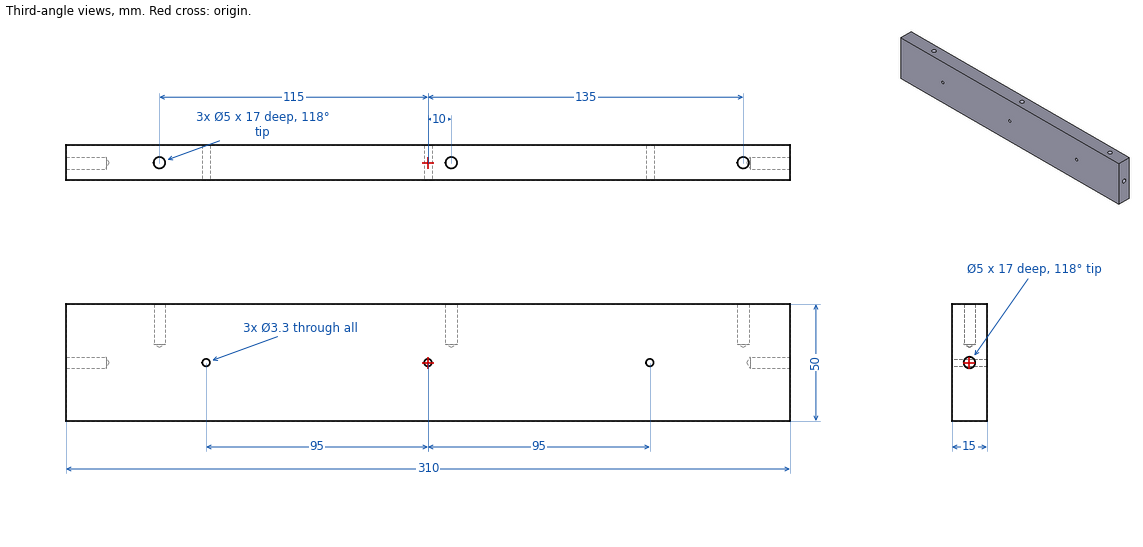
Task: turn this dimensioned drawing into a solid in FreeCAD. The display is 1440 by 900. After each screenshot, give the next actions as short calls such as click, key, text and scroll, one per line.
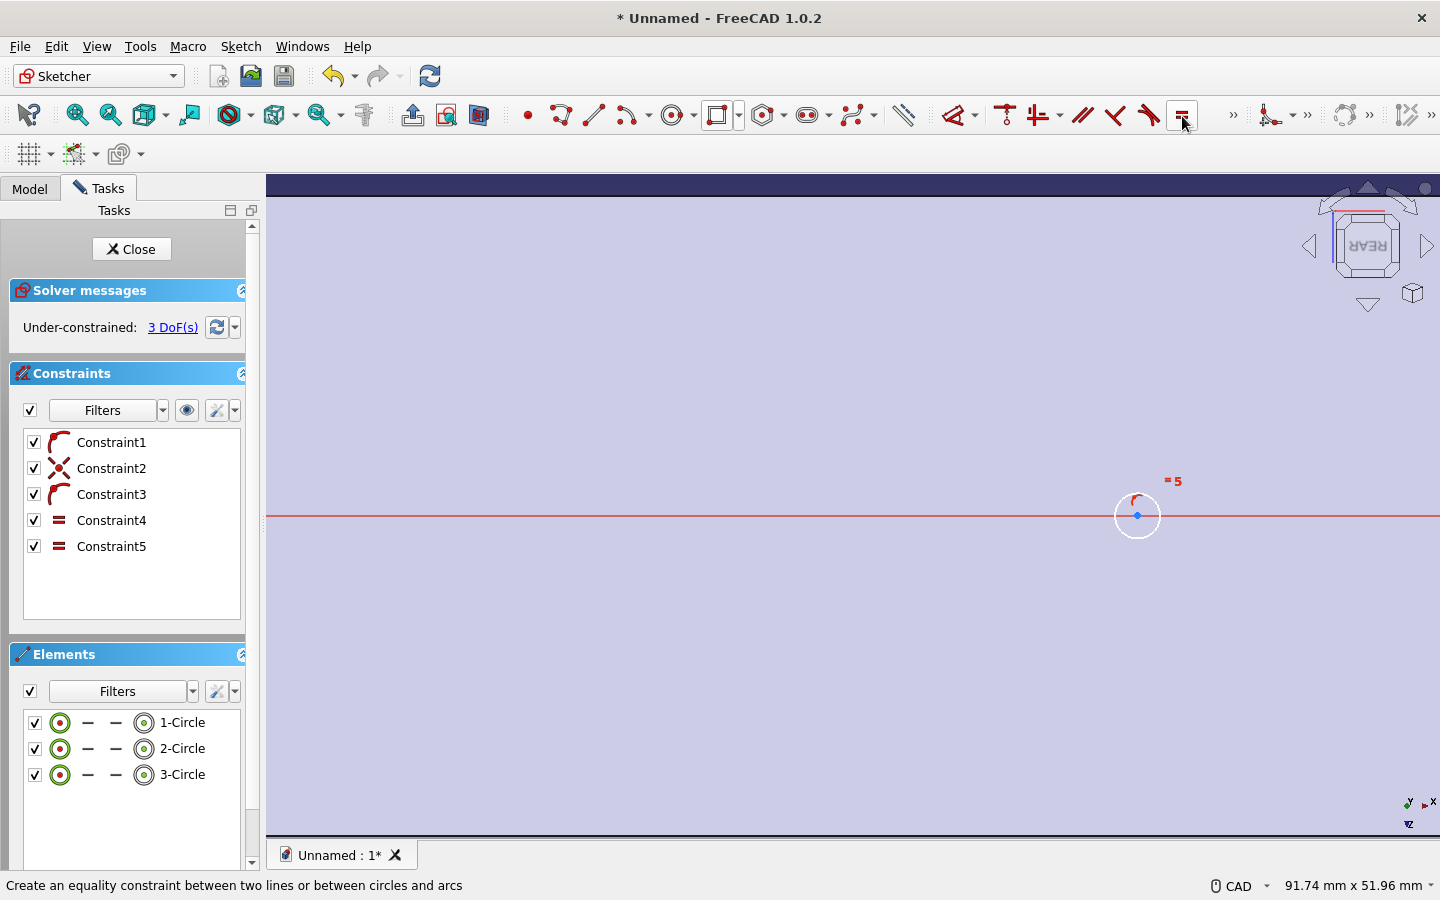
click(952, 116)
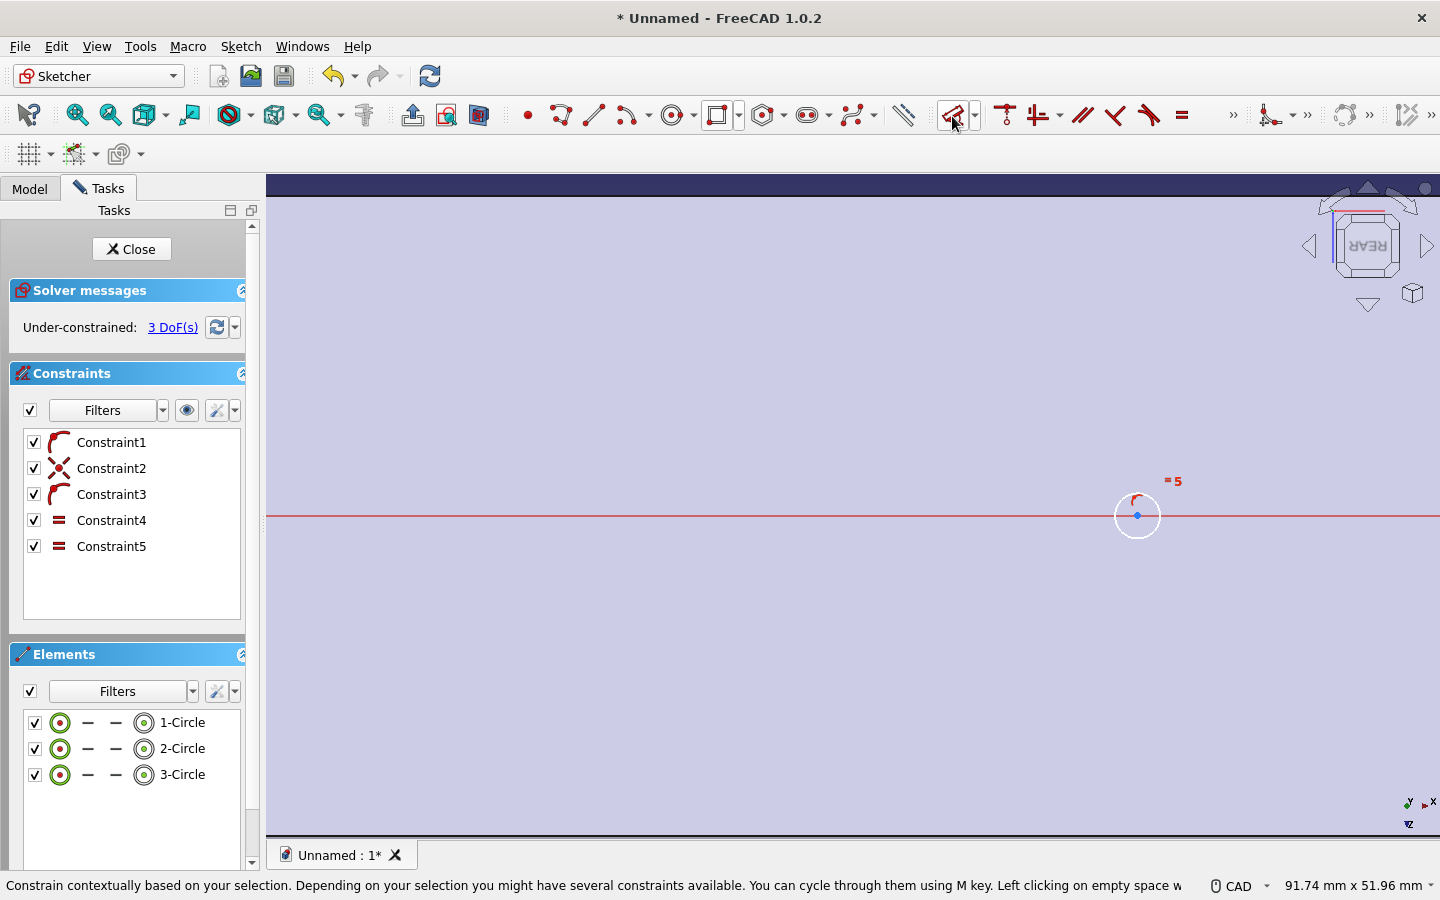
scroll(1156, 502, down, 6)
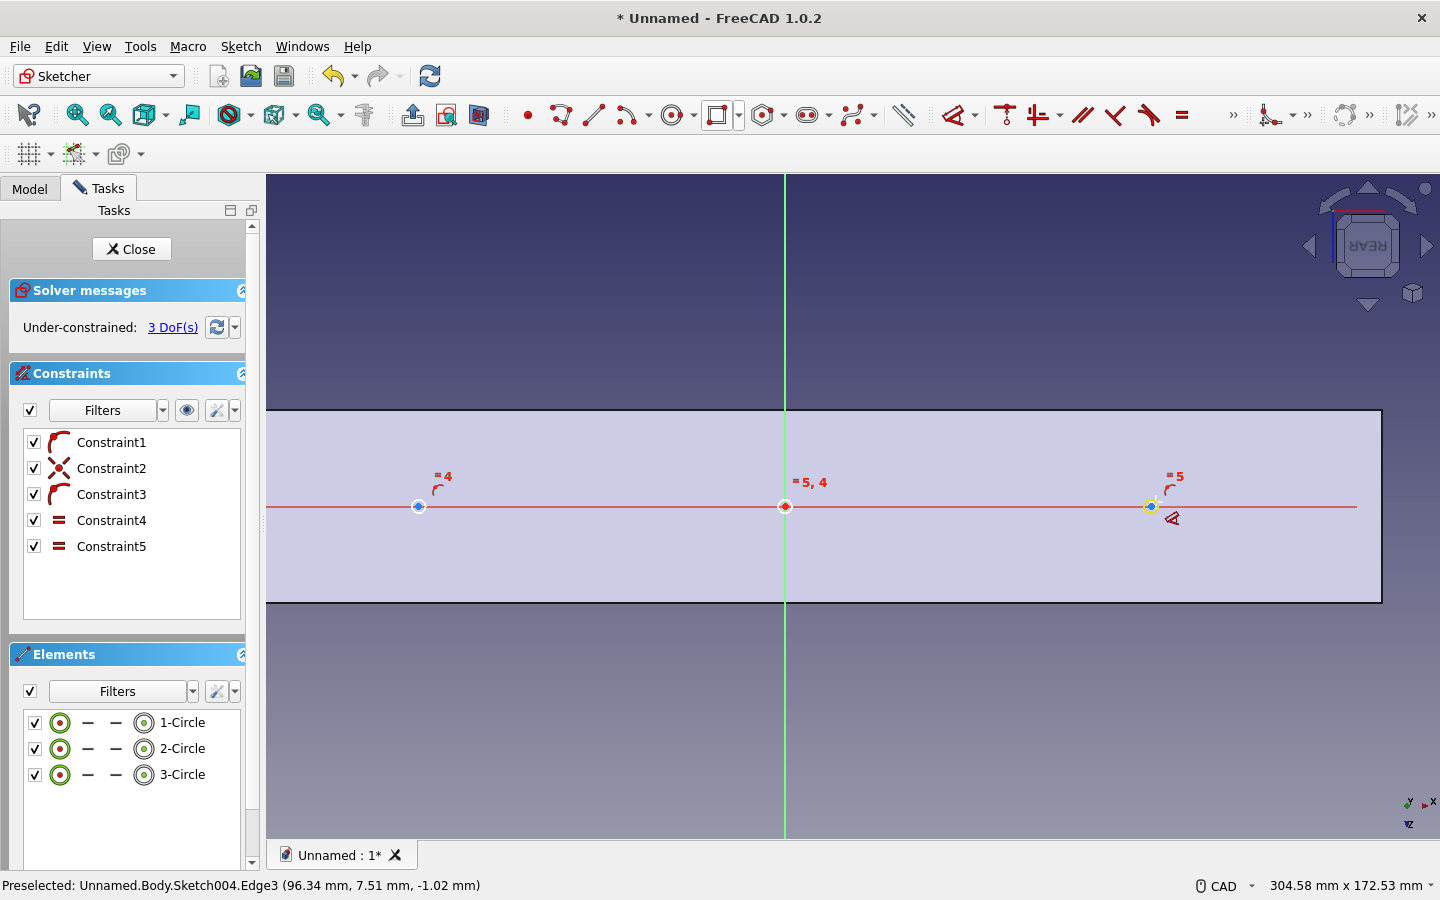
scroll(424, 502, up, 6)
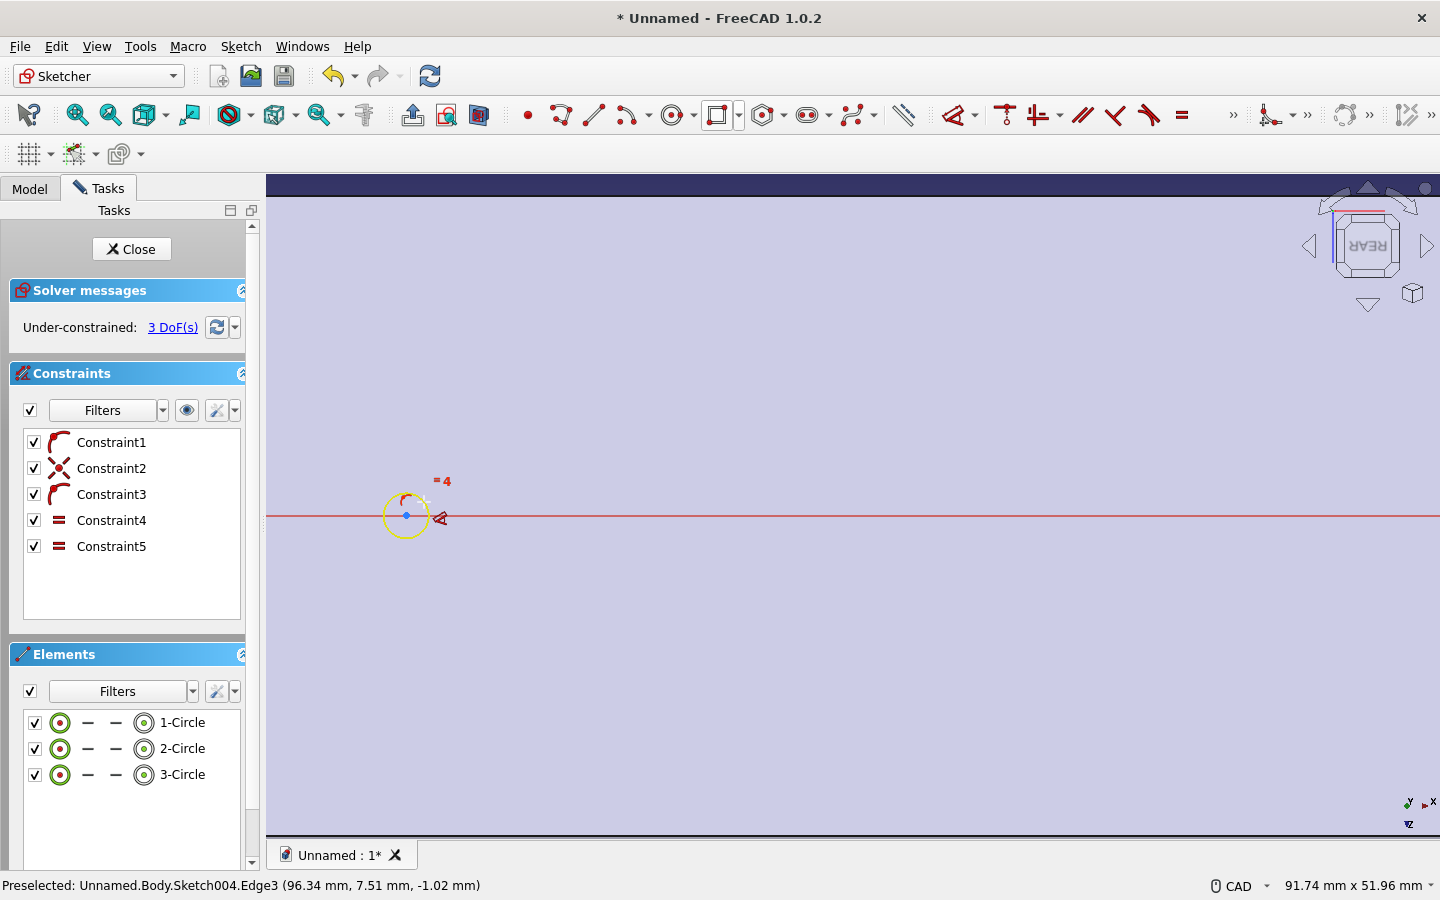
click(422, 500)
click(444, 477)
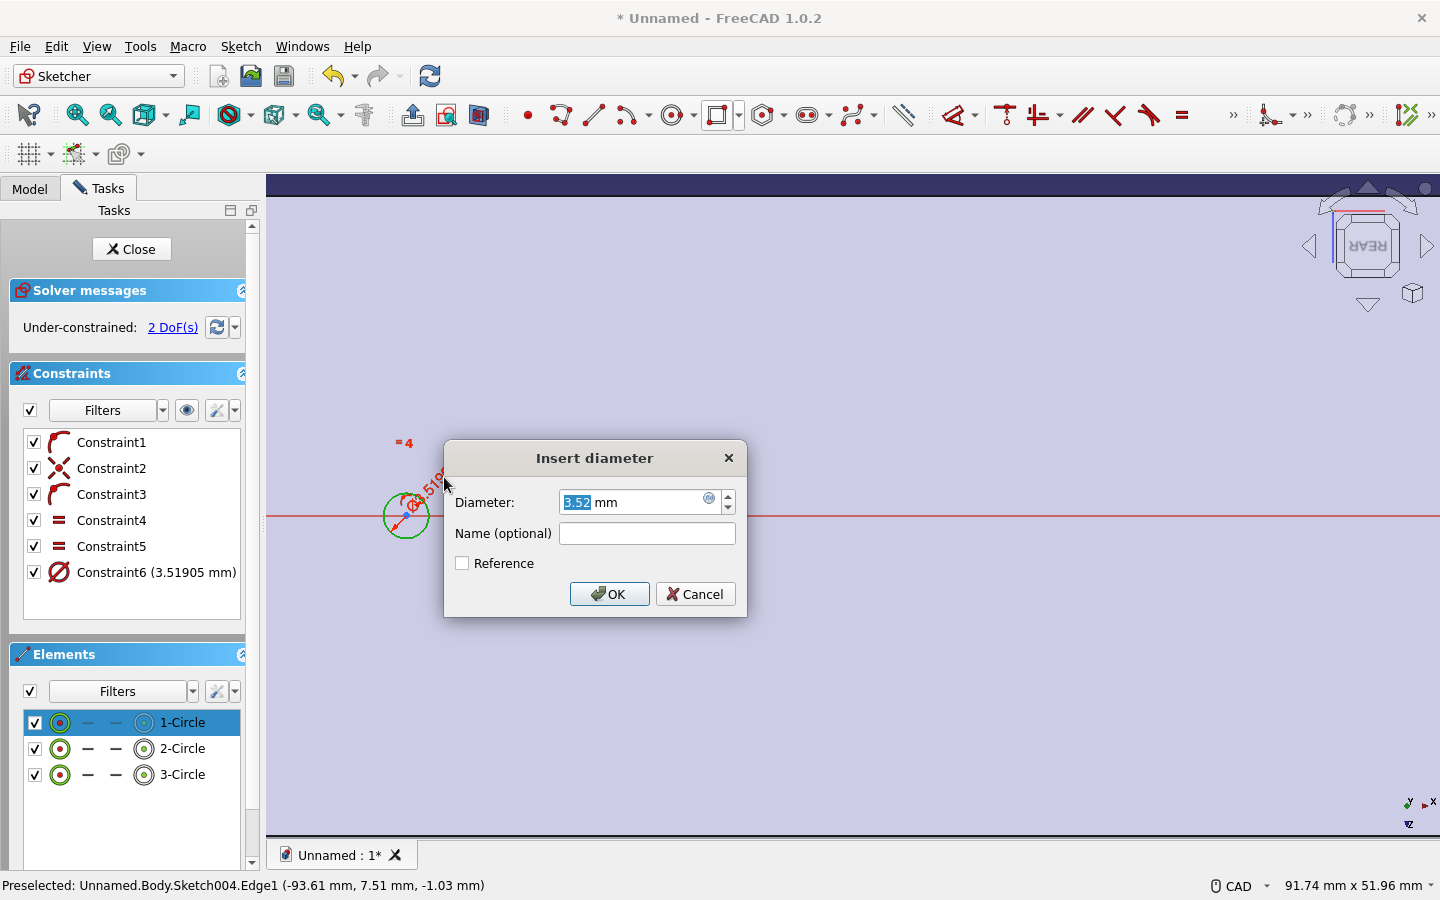
text(3.3)
key(Return)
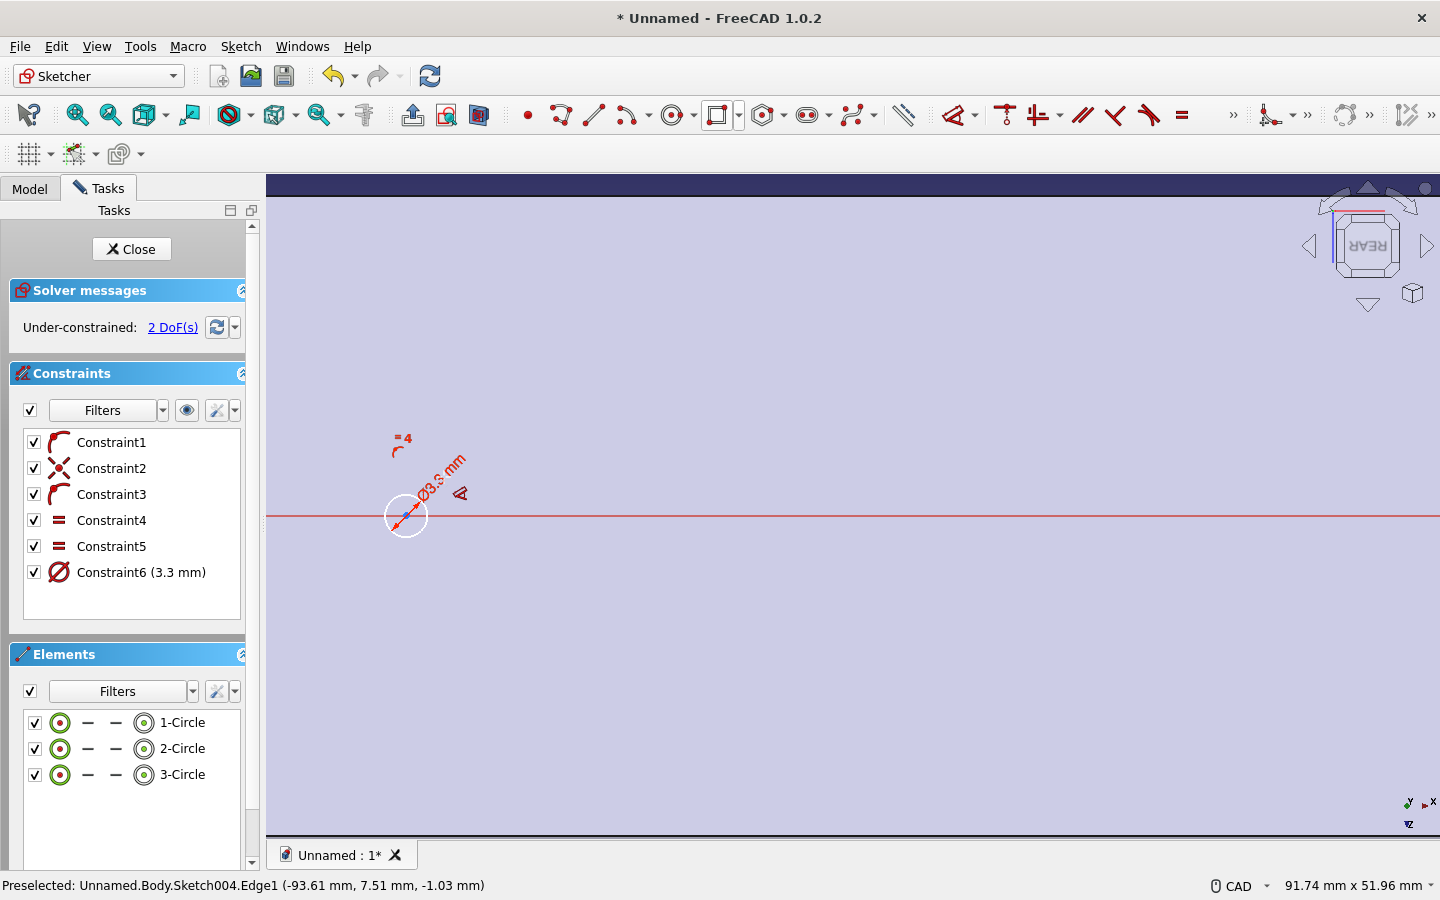
click(406, 516)
click(841, 550)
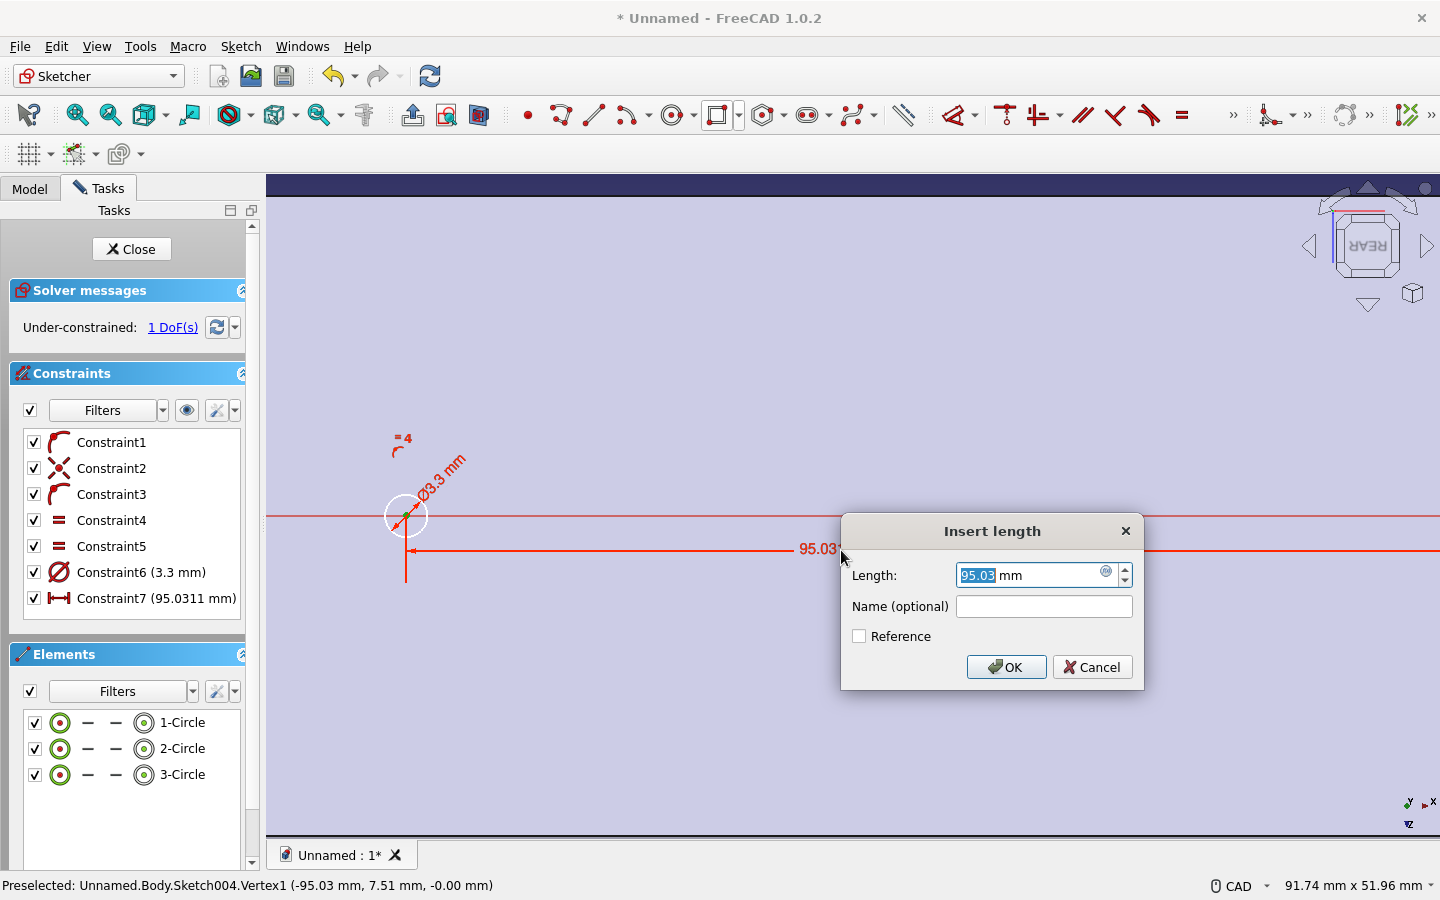
text(95)
key(Return)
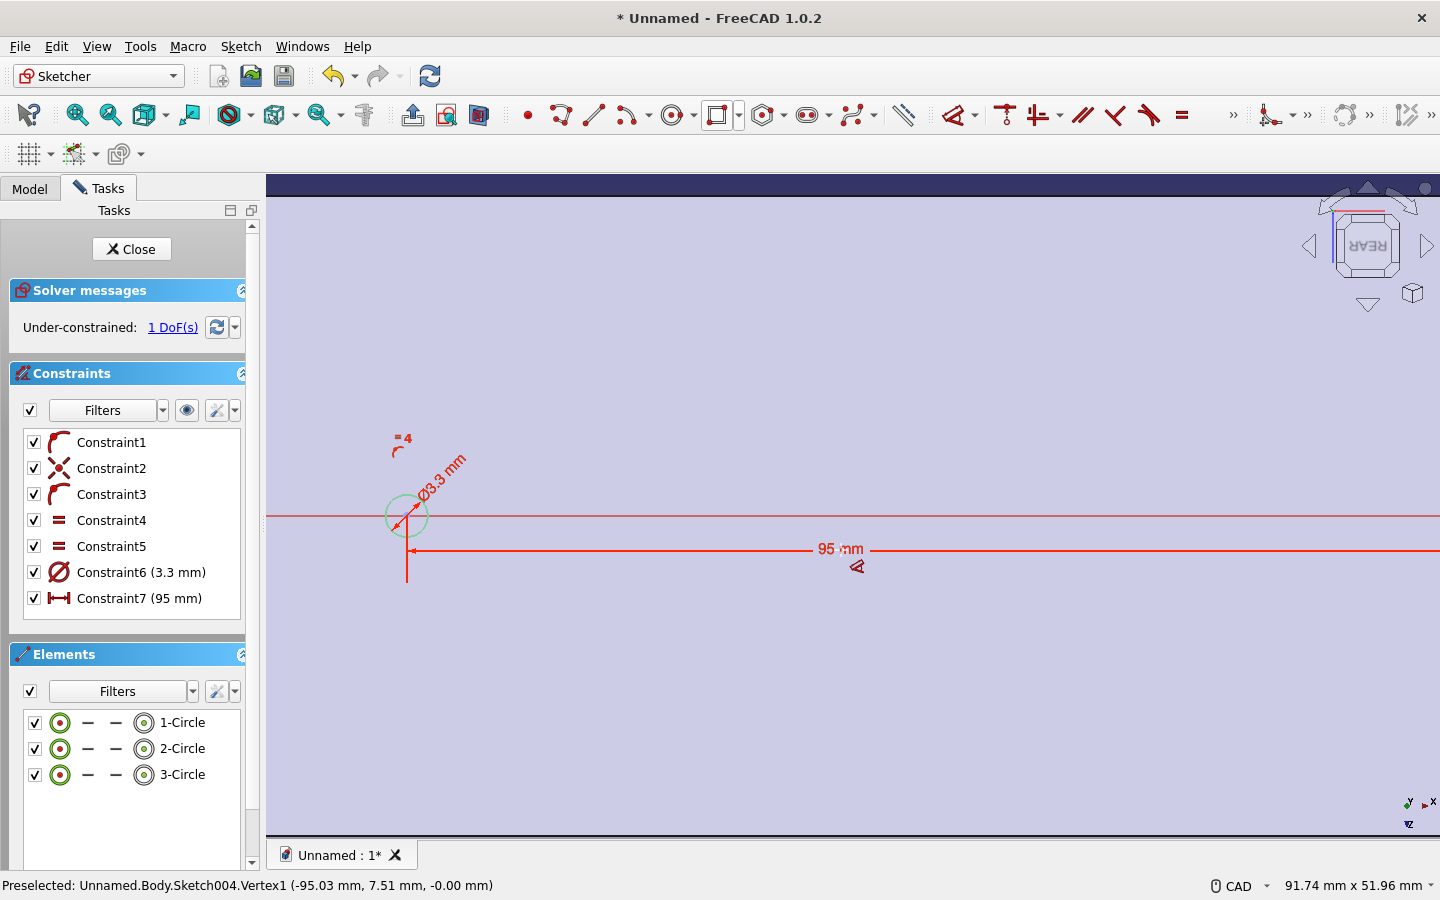
scroll(423, 502, down, 6)